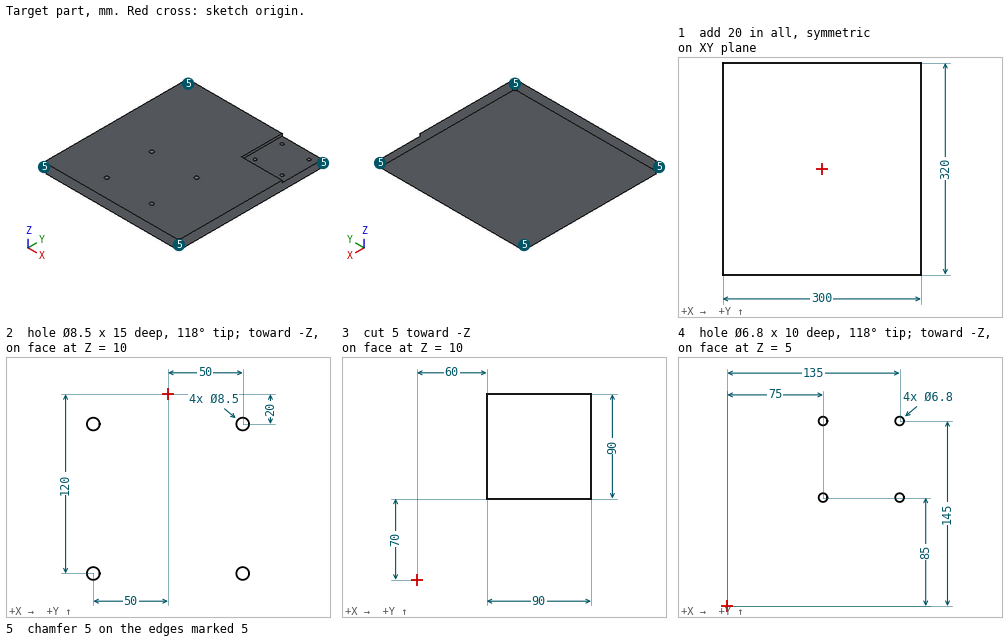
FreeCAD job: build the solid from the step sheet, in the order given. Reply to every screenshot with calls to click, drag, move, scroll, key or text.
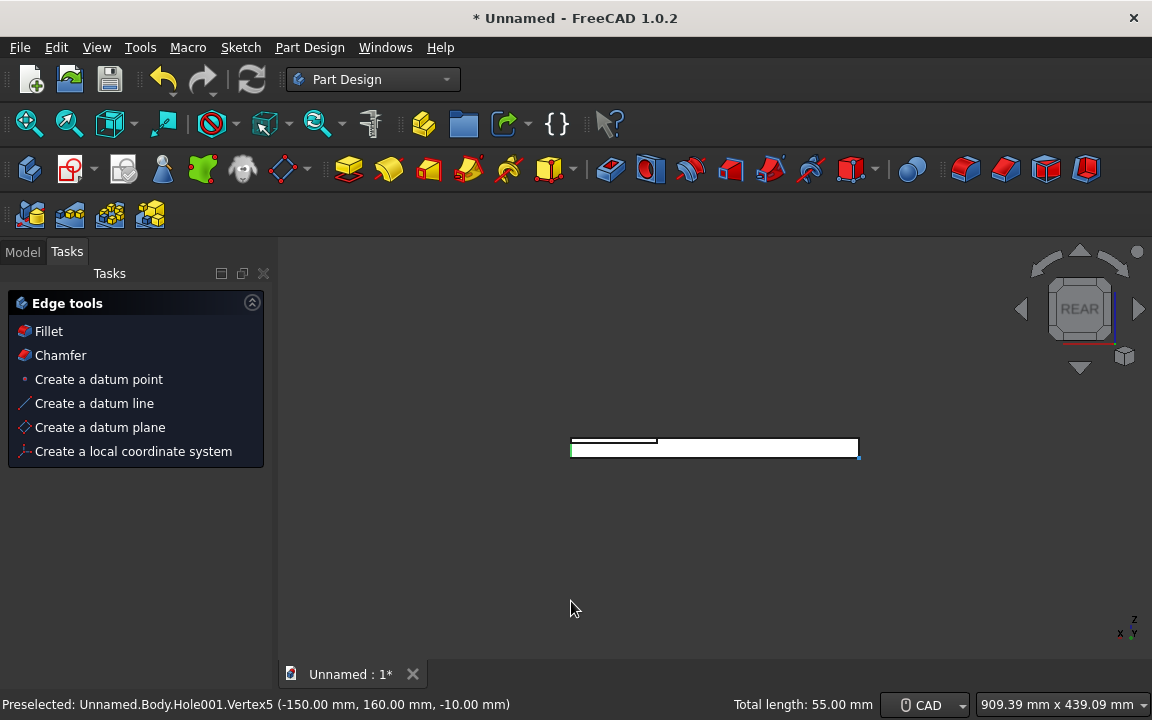
click(30, 124)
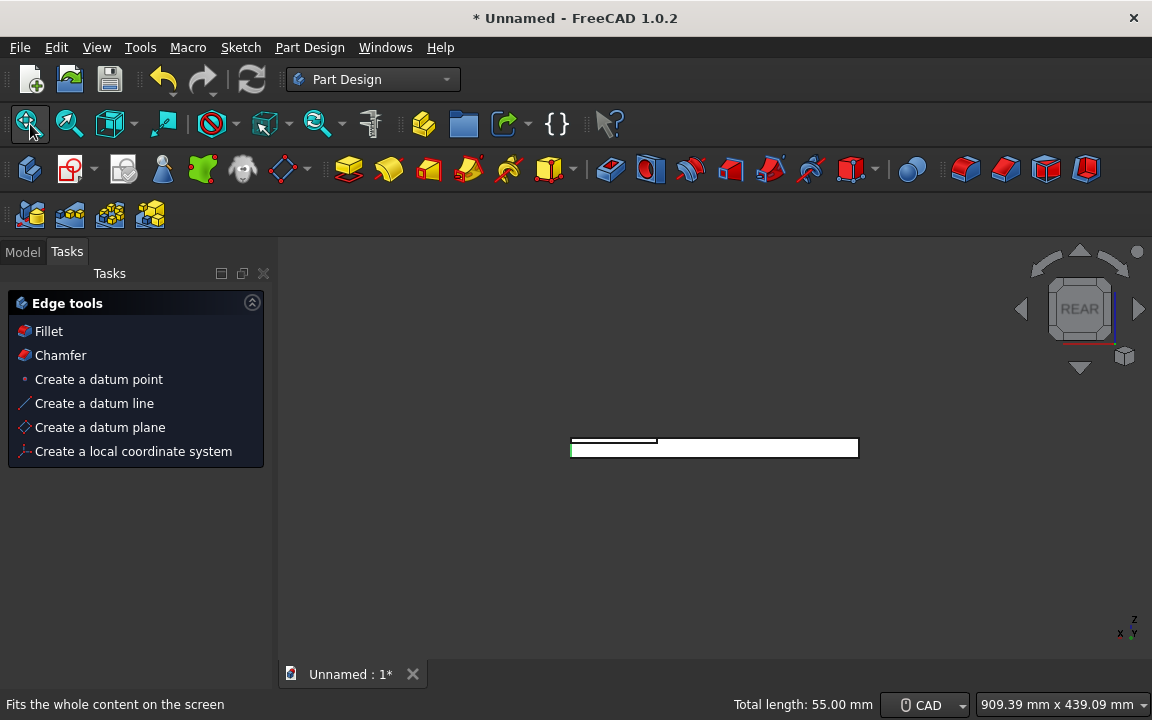
click(859, 447, ctrl)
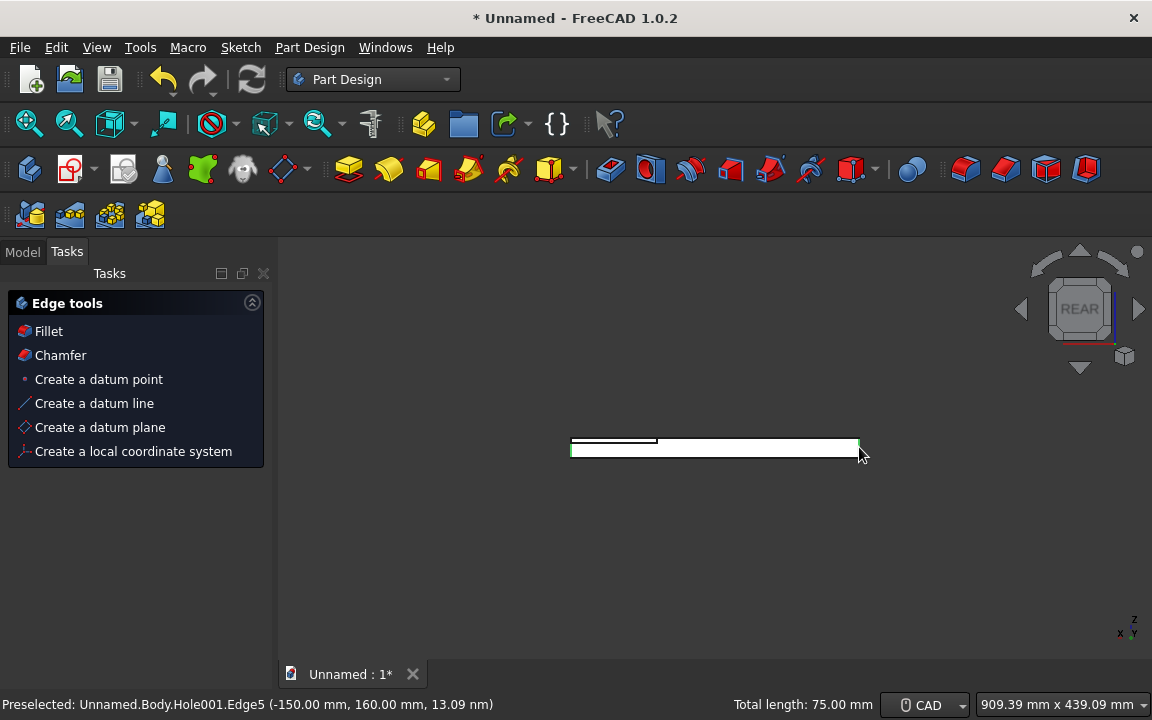
click(1006, 170)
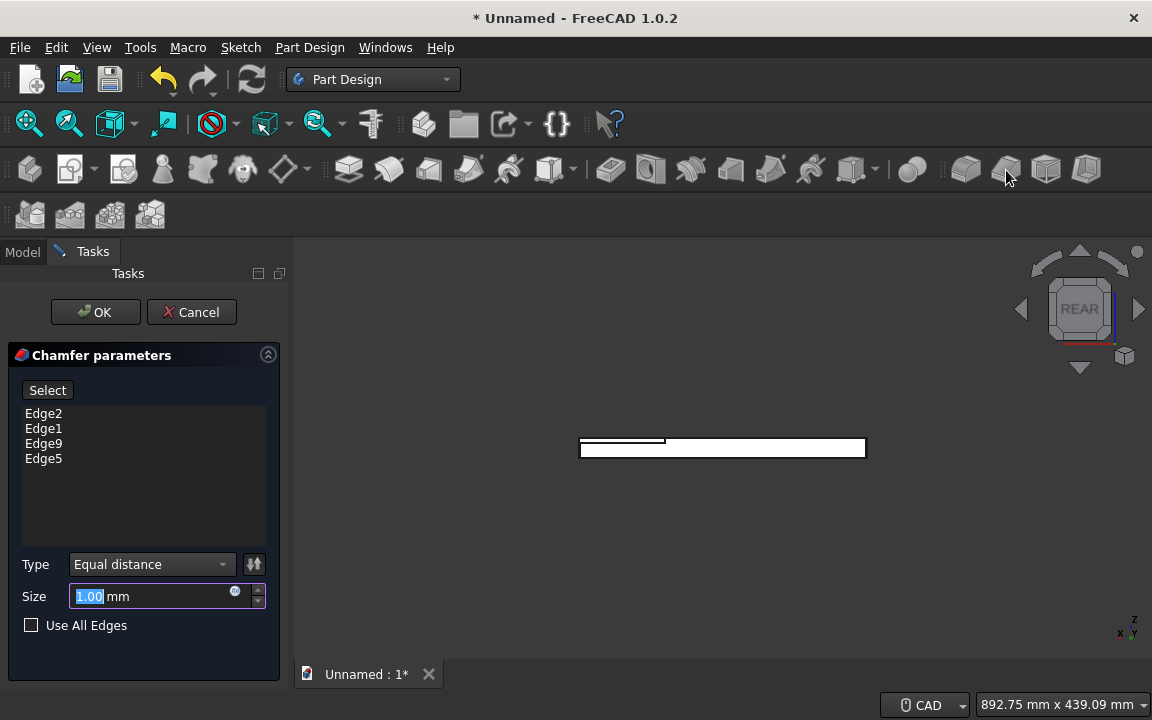
text(5)
key(Tab)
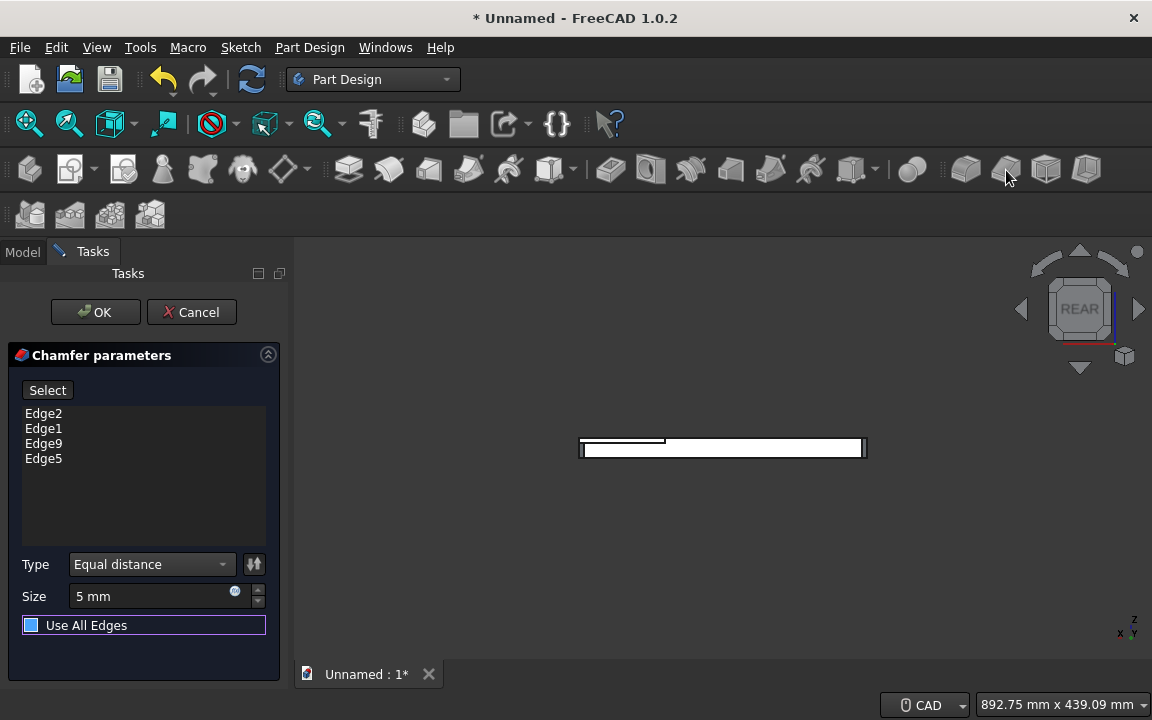
click(96, 312)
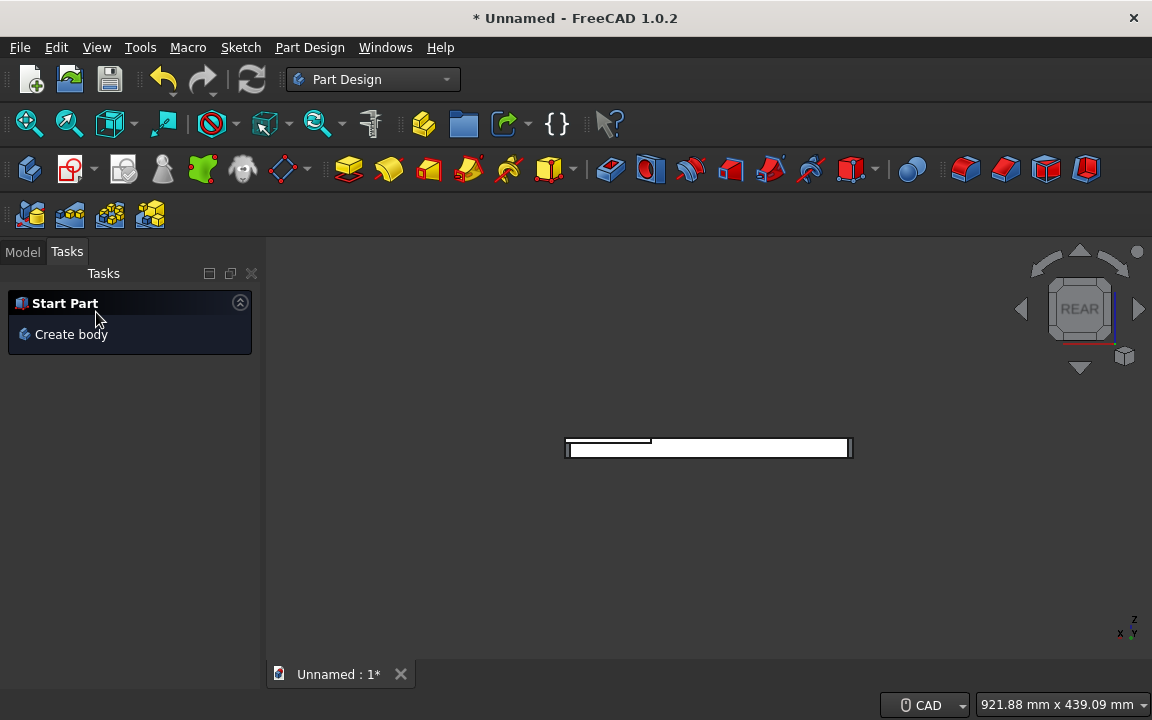
key(0)